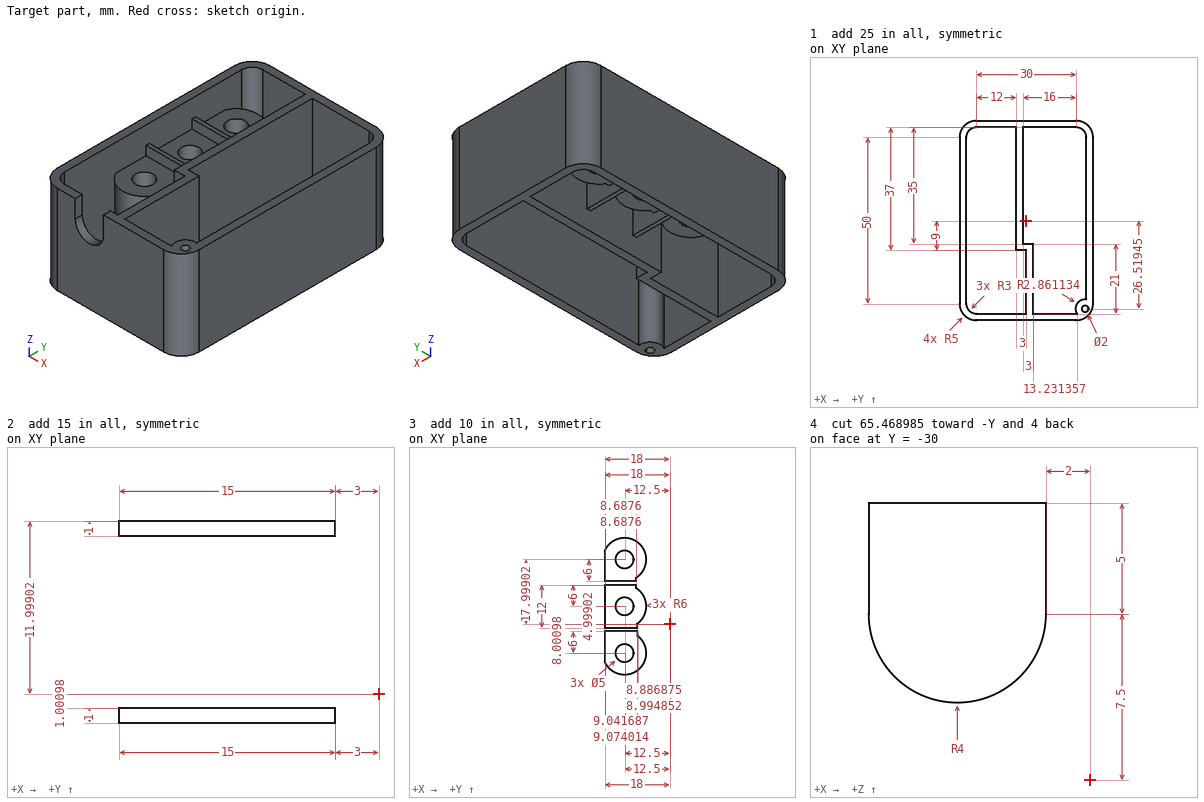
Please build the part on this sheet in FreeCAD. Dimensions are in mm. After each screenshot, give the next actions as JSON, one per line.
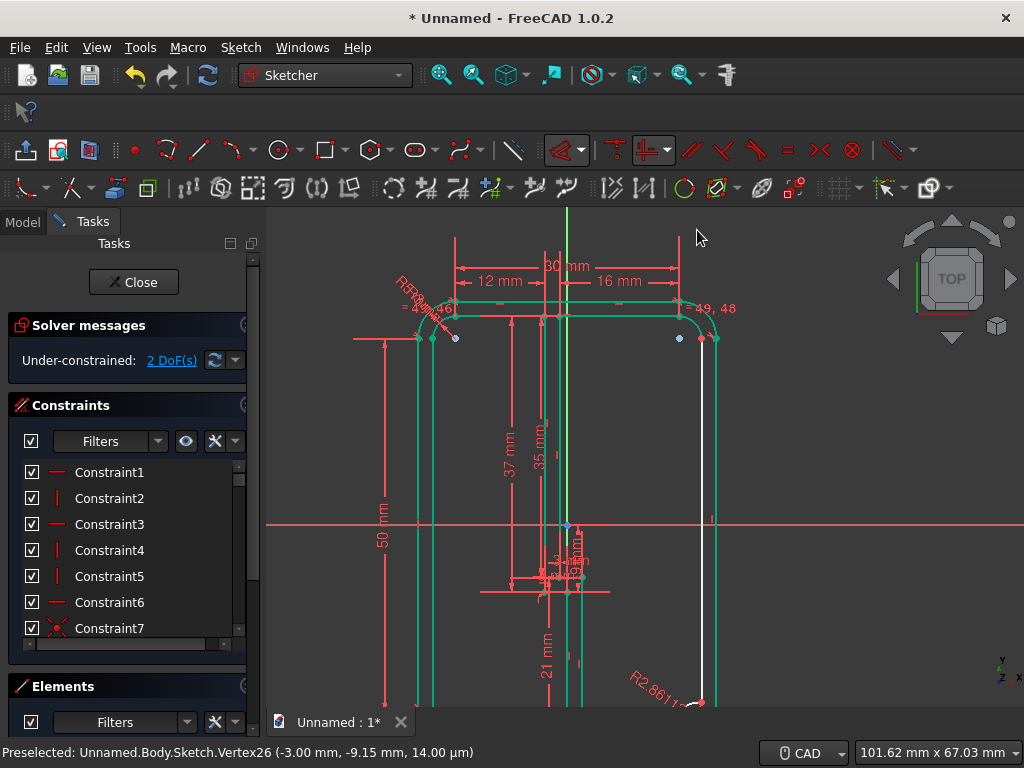
{"action": "scroll", "coordinate": [595, 318], "scroll_direction": "down", "scroll_amount": 2}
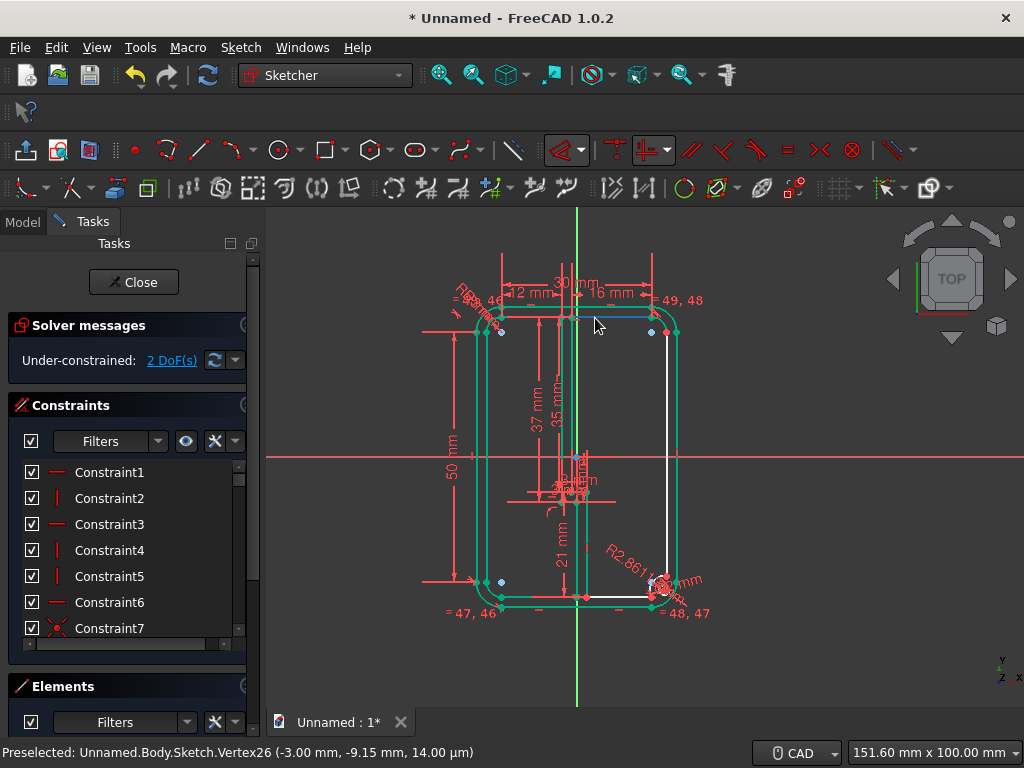
{"action": "left_click", "coordinate": [664, 590]}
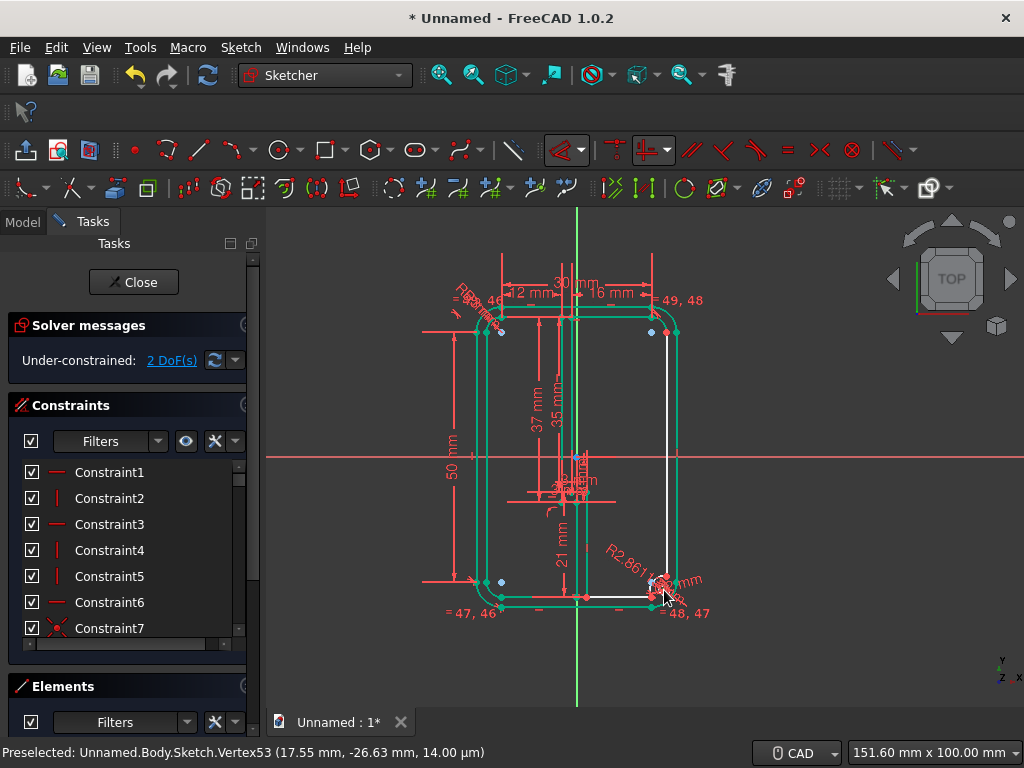
{"action": "key", "text": "i"}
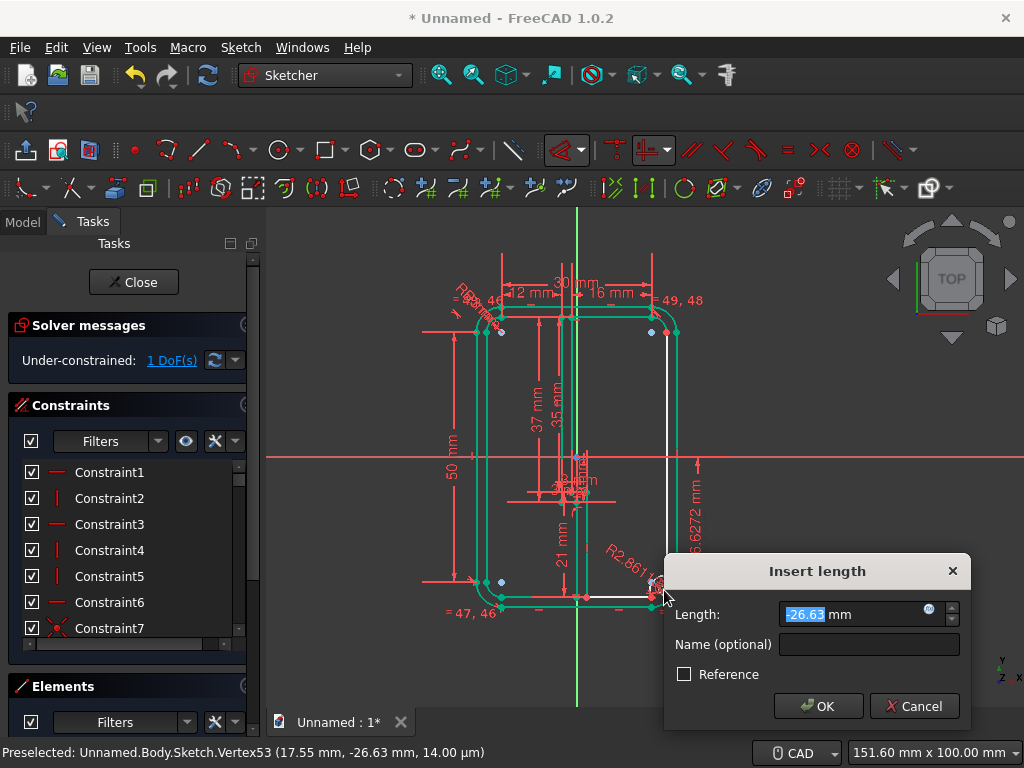
{"action": "type", "text": "-26.51945"}
{"action": "key", "text": "Return"}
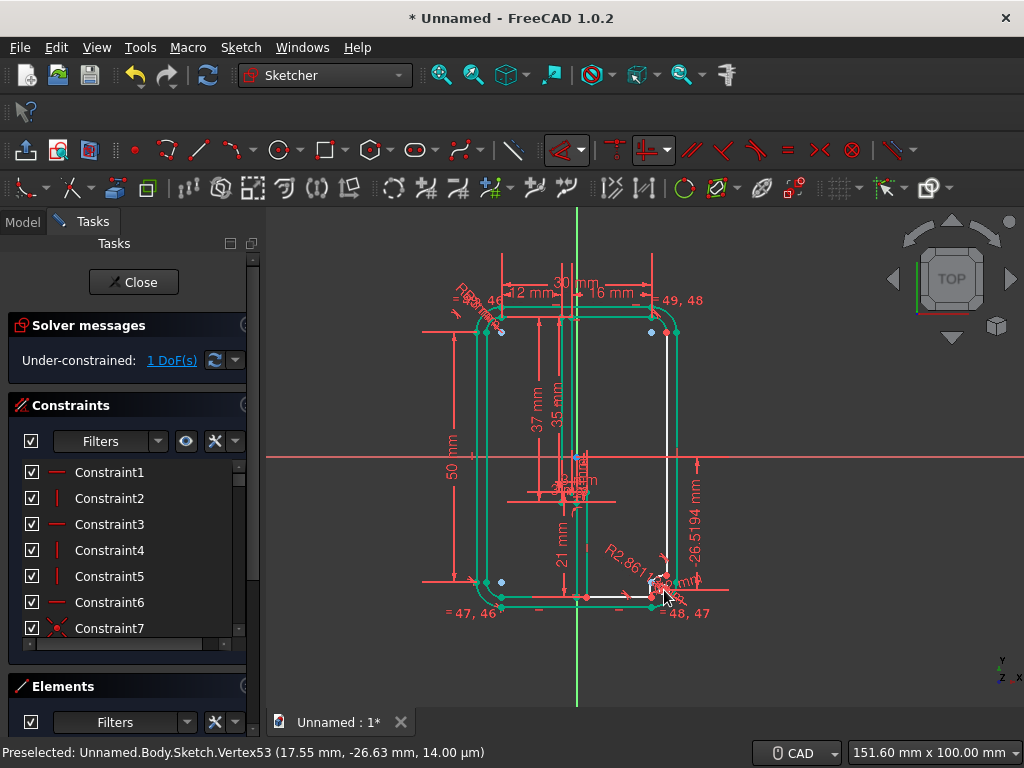
{"action": "scroll", "coordinate": [632, 597], "scroll_direction": "up", "scroll_amount": 2}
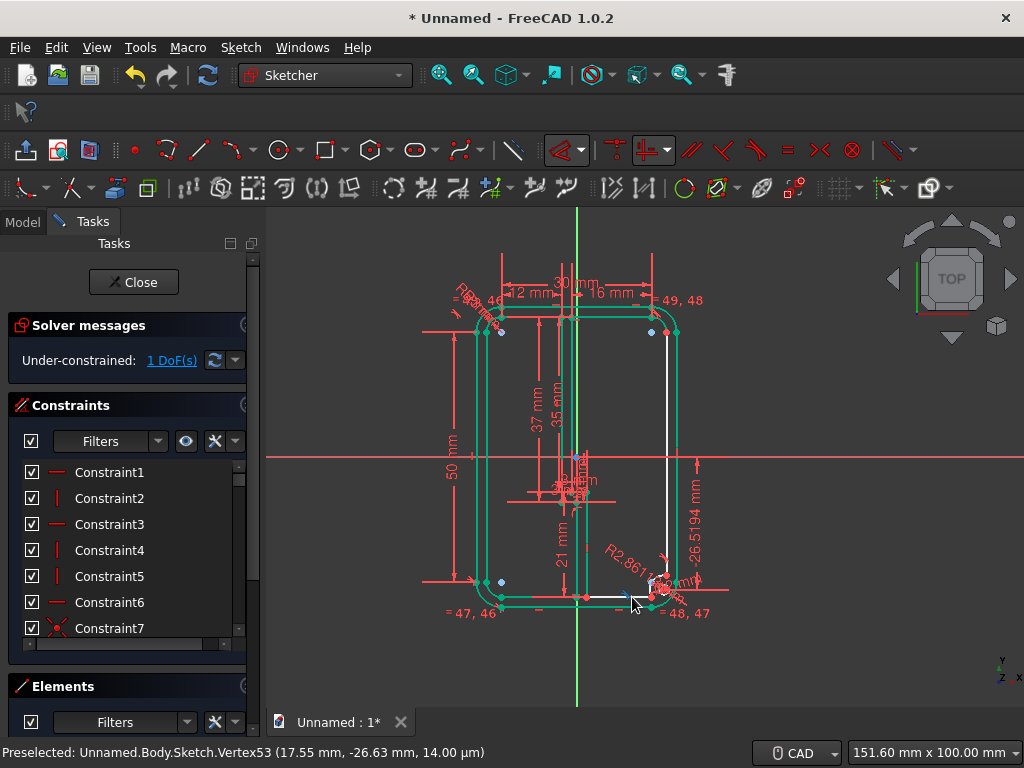
{"action": "left_click", "coordinate": [593, 597]}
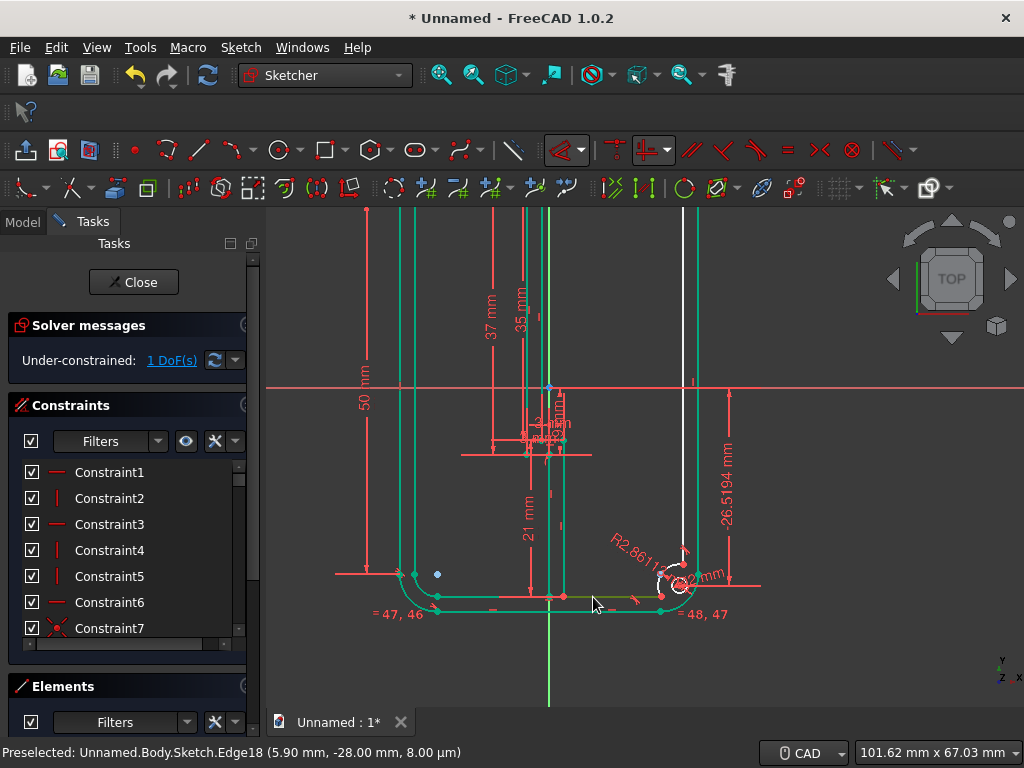
{"action": "left_click", "coordinate": [584, 150]}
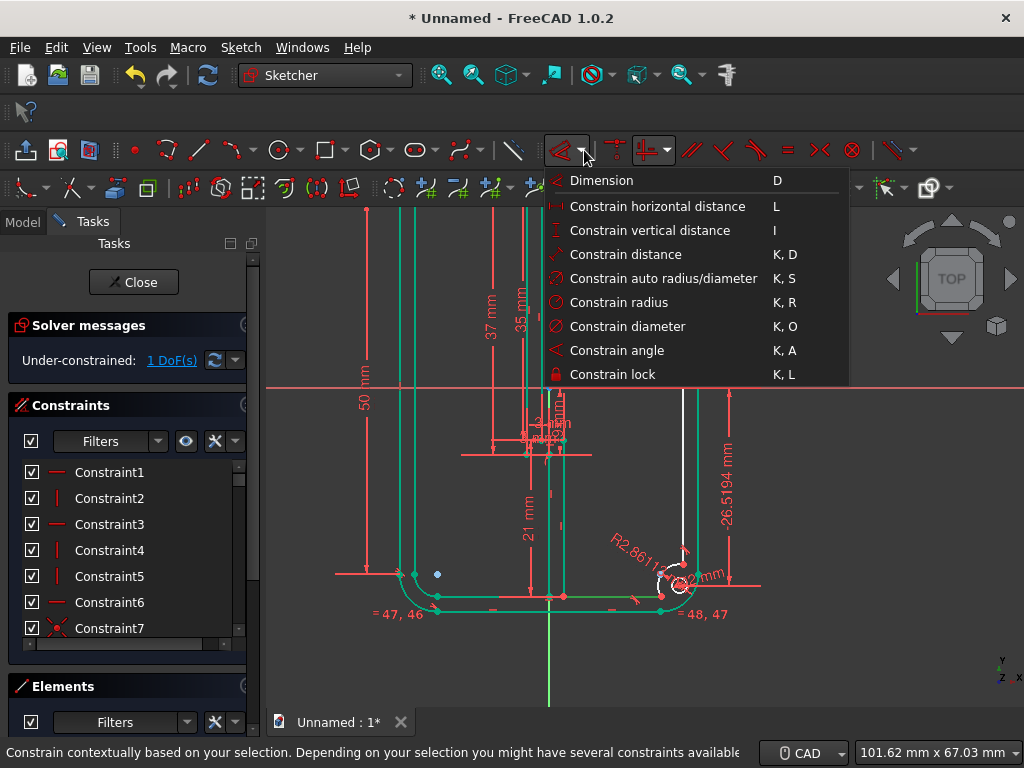
{"action": "left_click", "coordinate": [697, 206]}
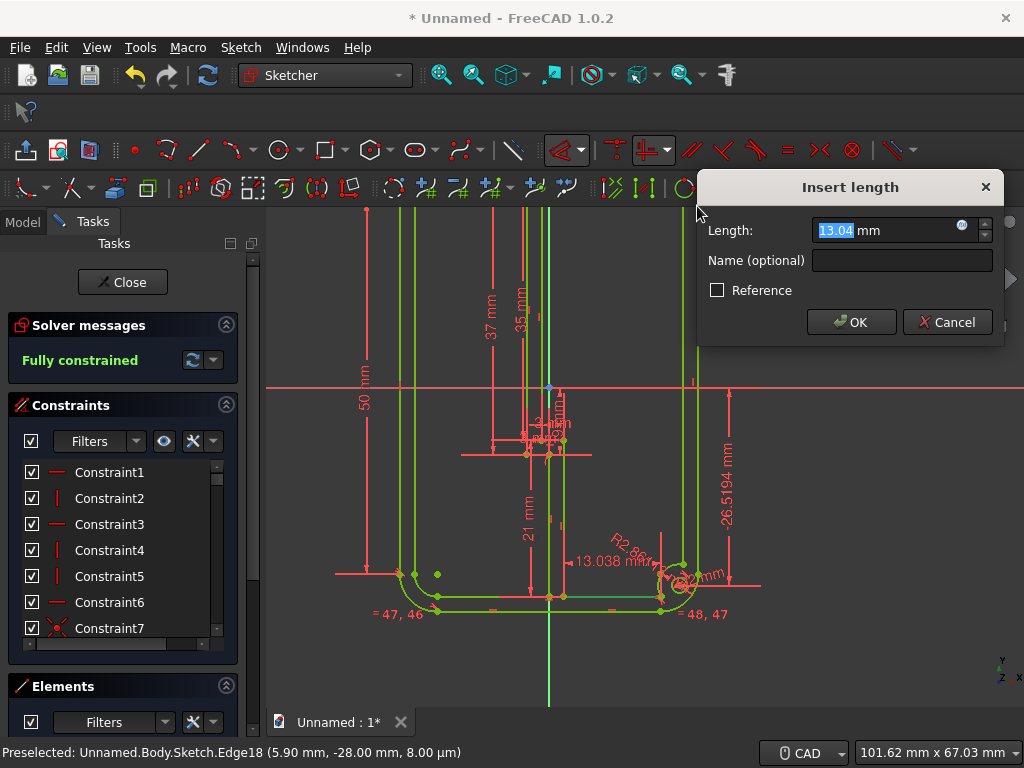
{"action": "type", "text": "13.231357"}
{"action": "key", "text": "Return"}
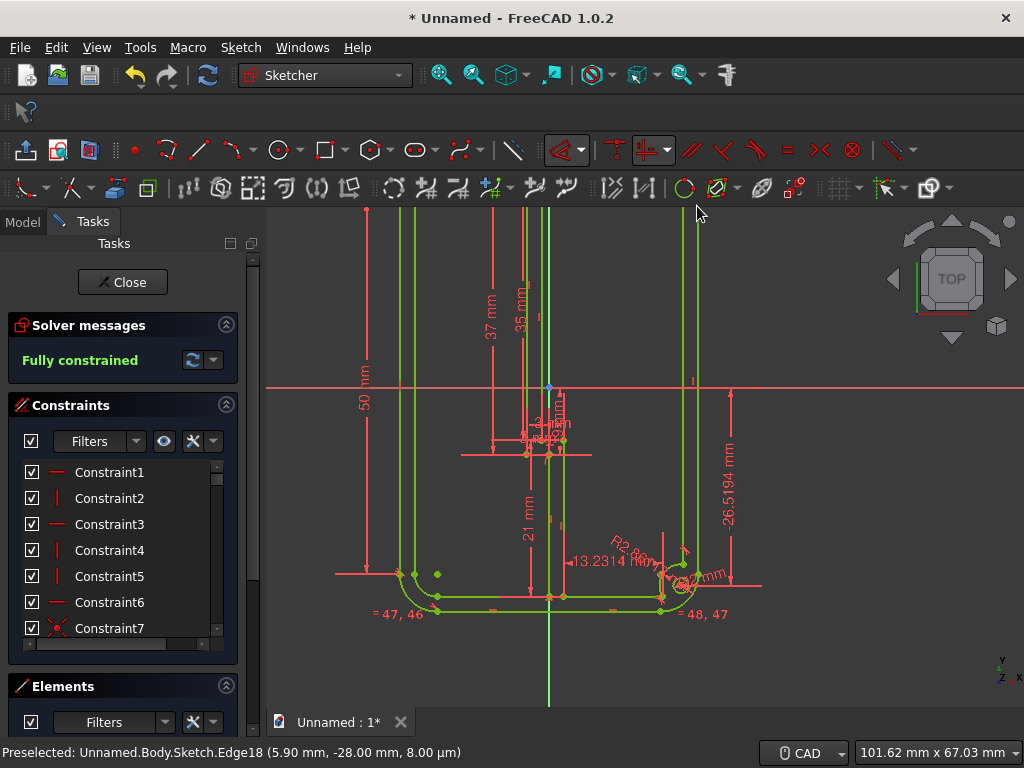
{"action": "left_click", "coordinate": [123, 282]}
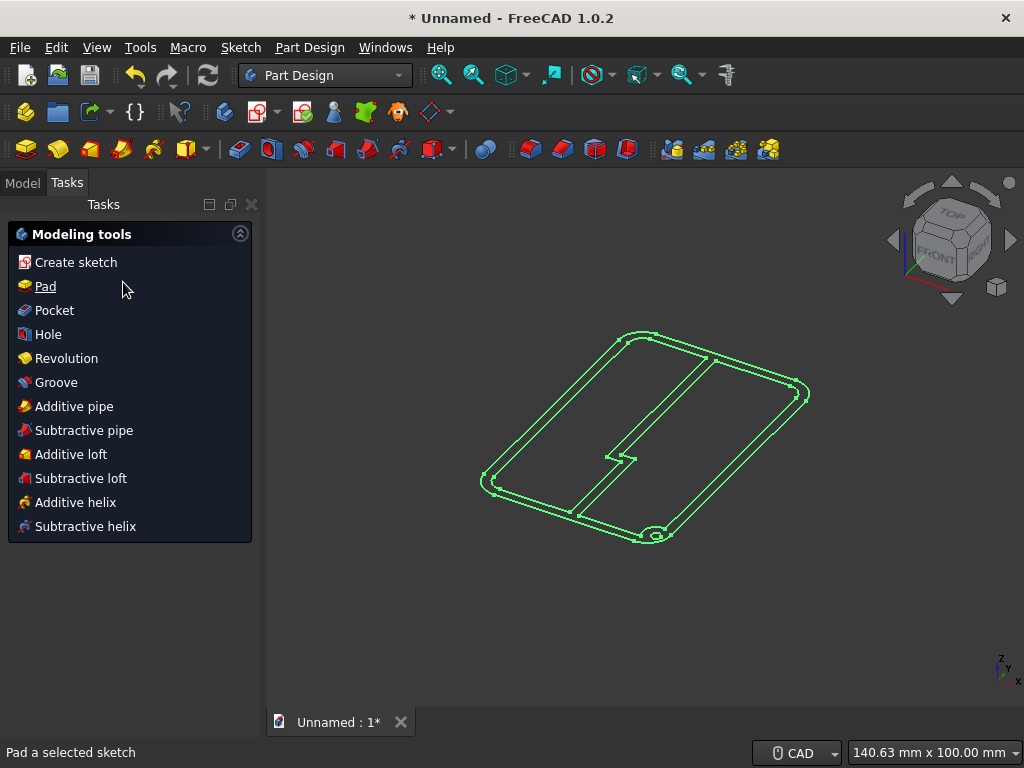
{"action": "left_click", "coordinate": [26, 150]}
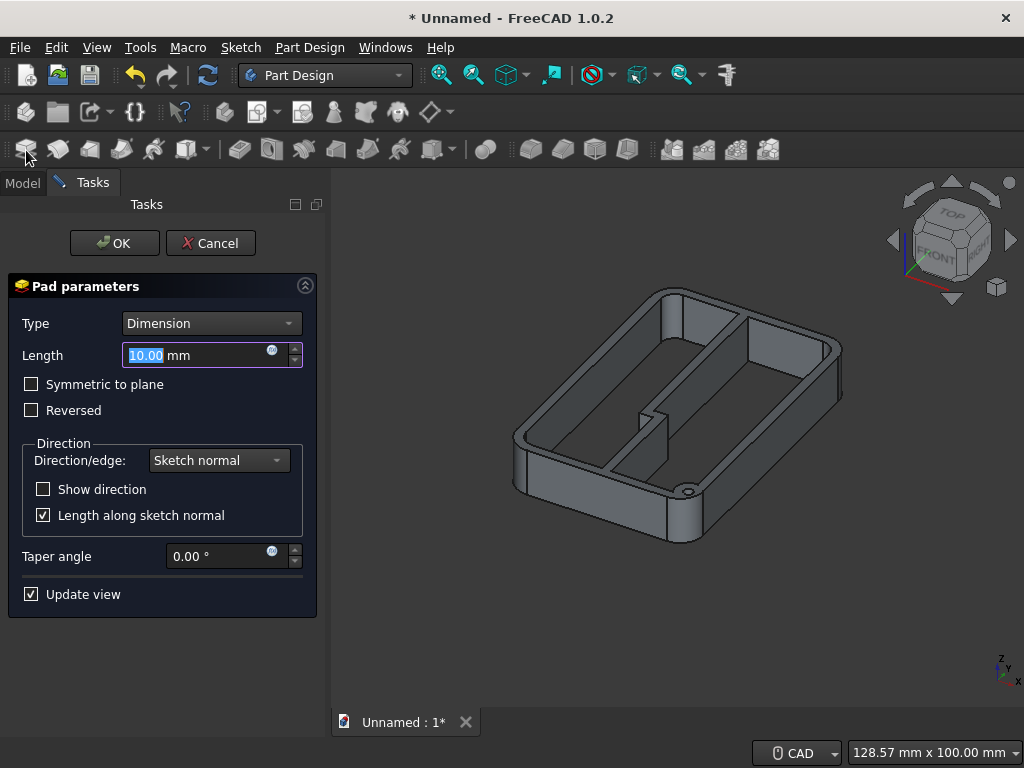
{"action": "type", "text": "25"}
{"action": "key", "text": "Tab"}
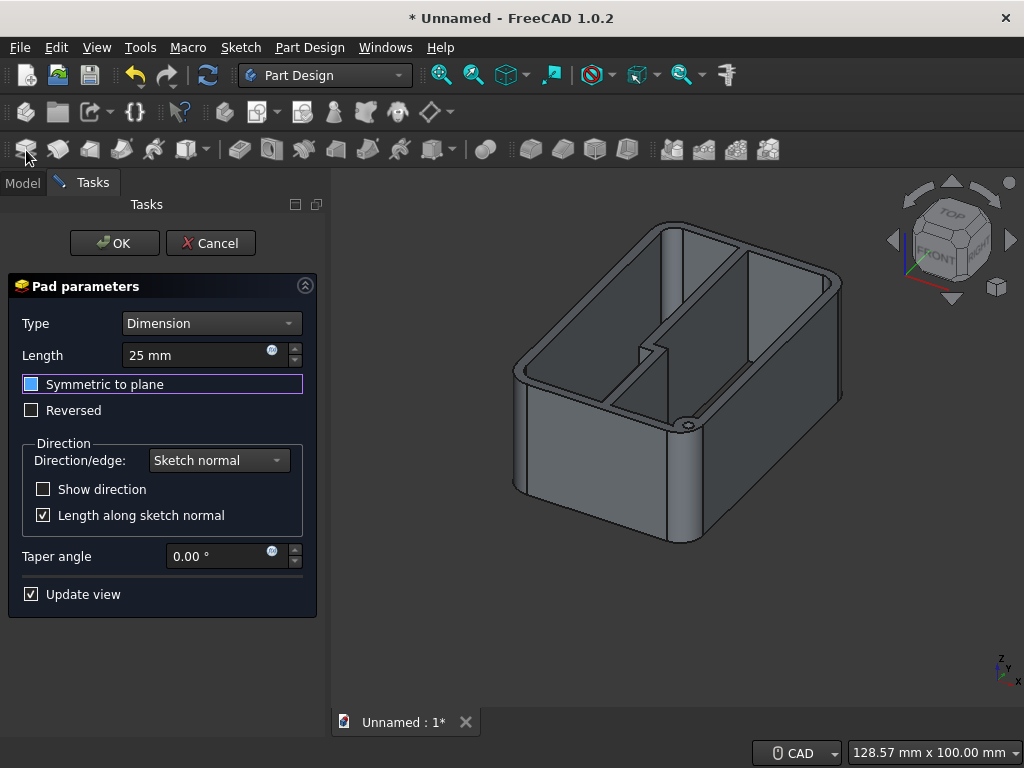
{"action": "left_click", "coordinate": [30, 384]}